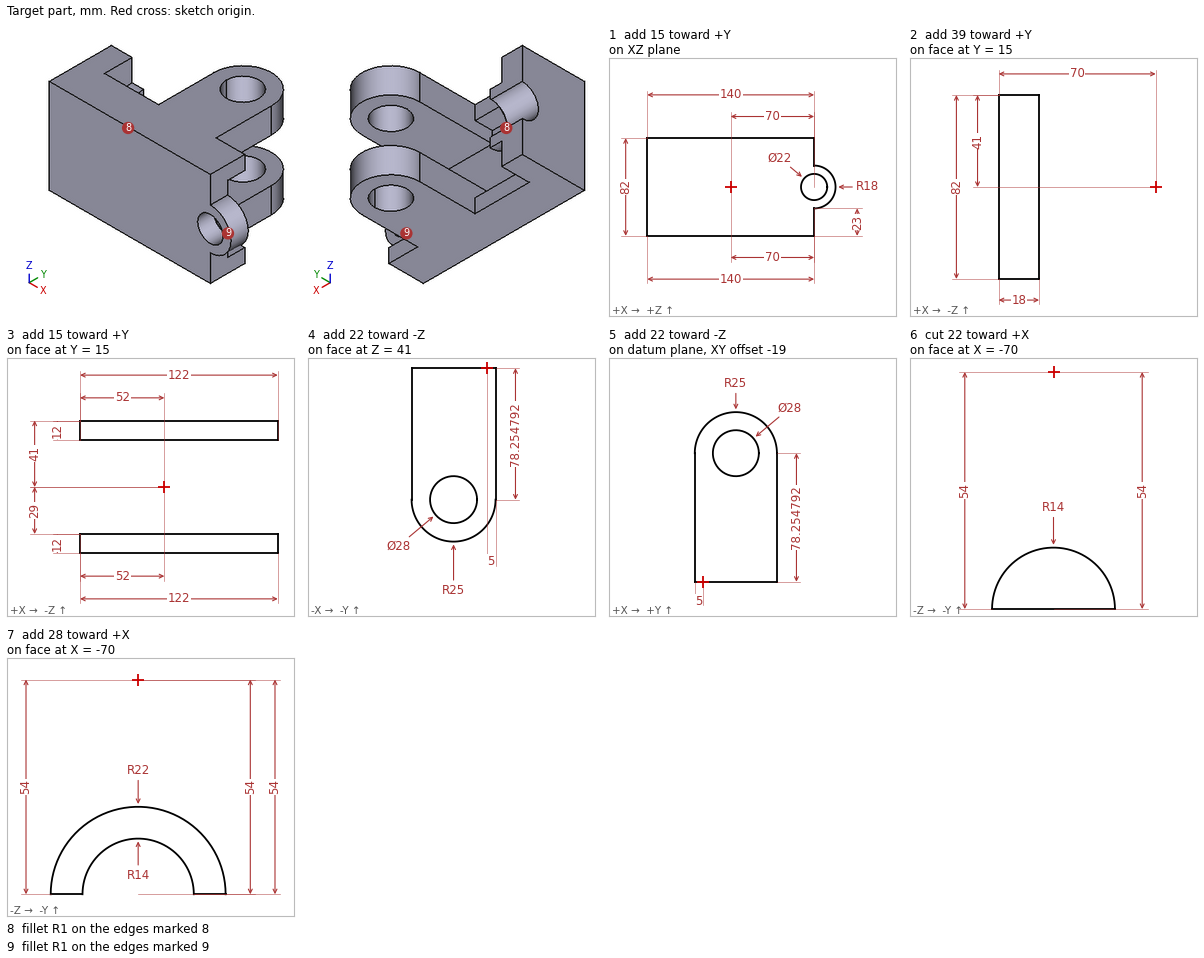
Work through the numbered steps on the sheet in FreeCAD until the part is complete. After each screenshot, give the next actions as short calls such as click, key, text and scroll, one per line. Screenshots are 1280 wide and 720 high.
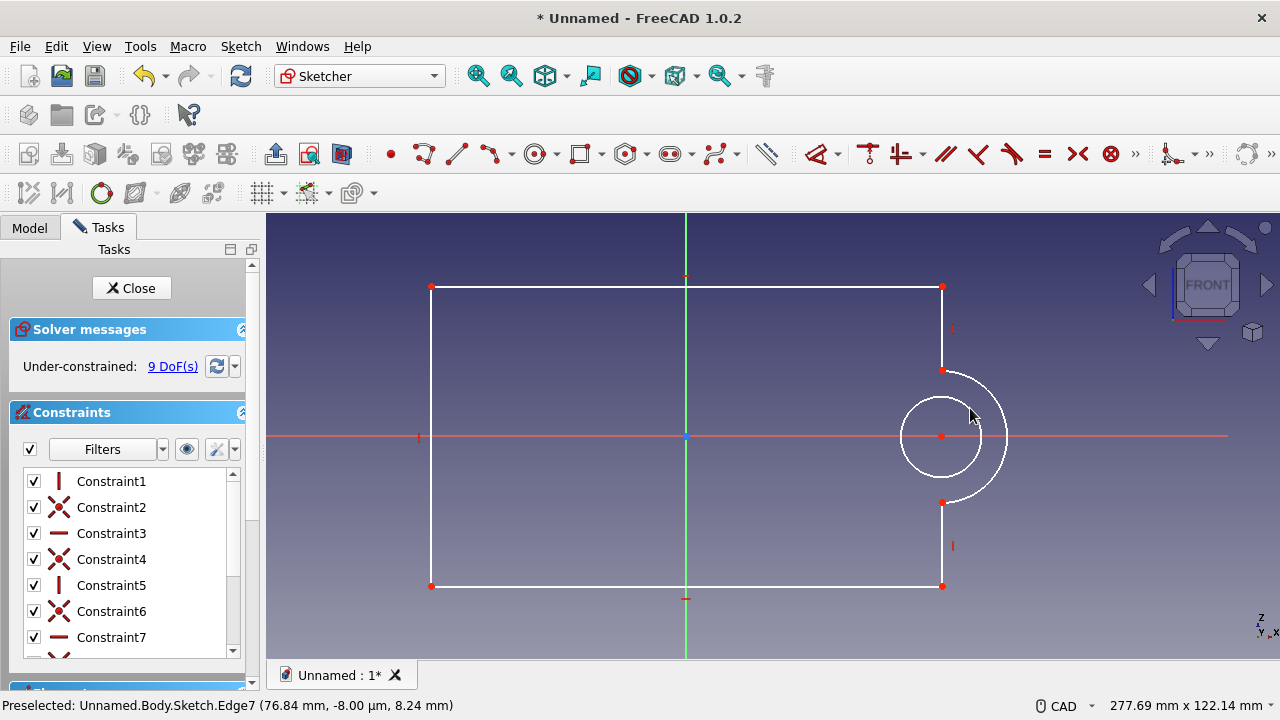
click(941, 437)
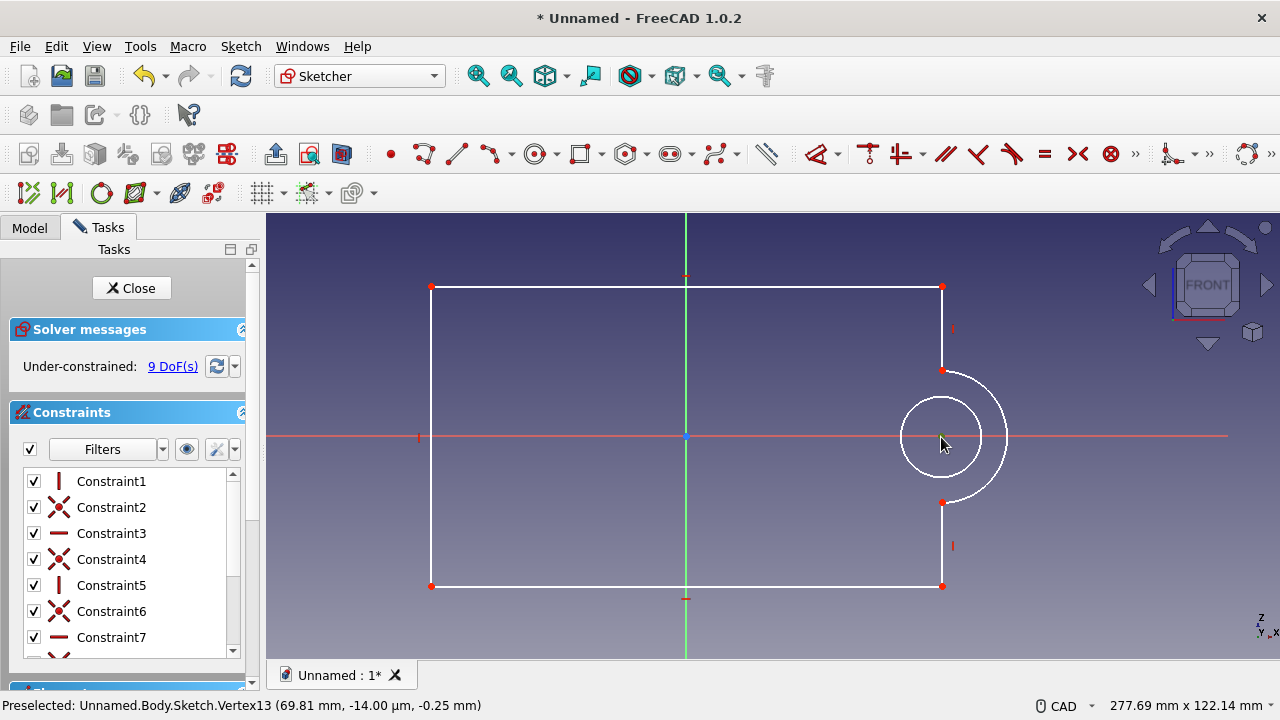
click(353, 436)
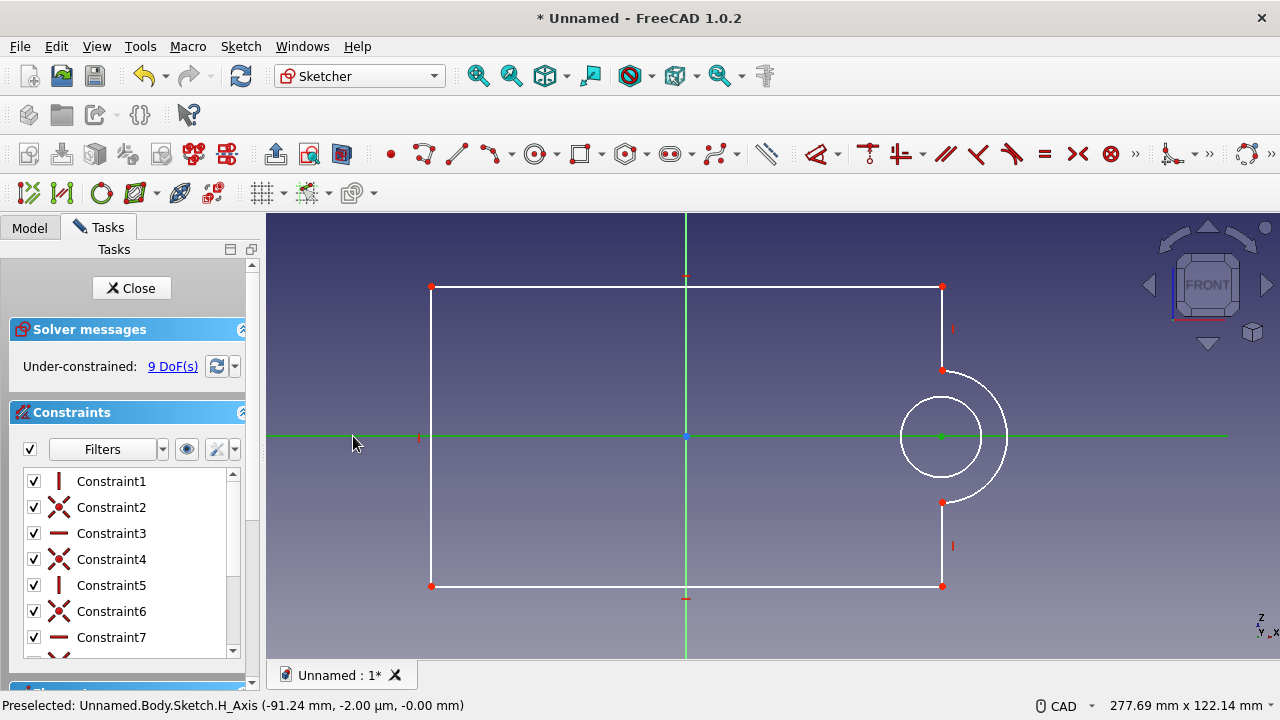
click(868, 154)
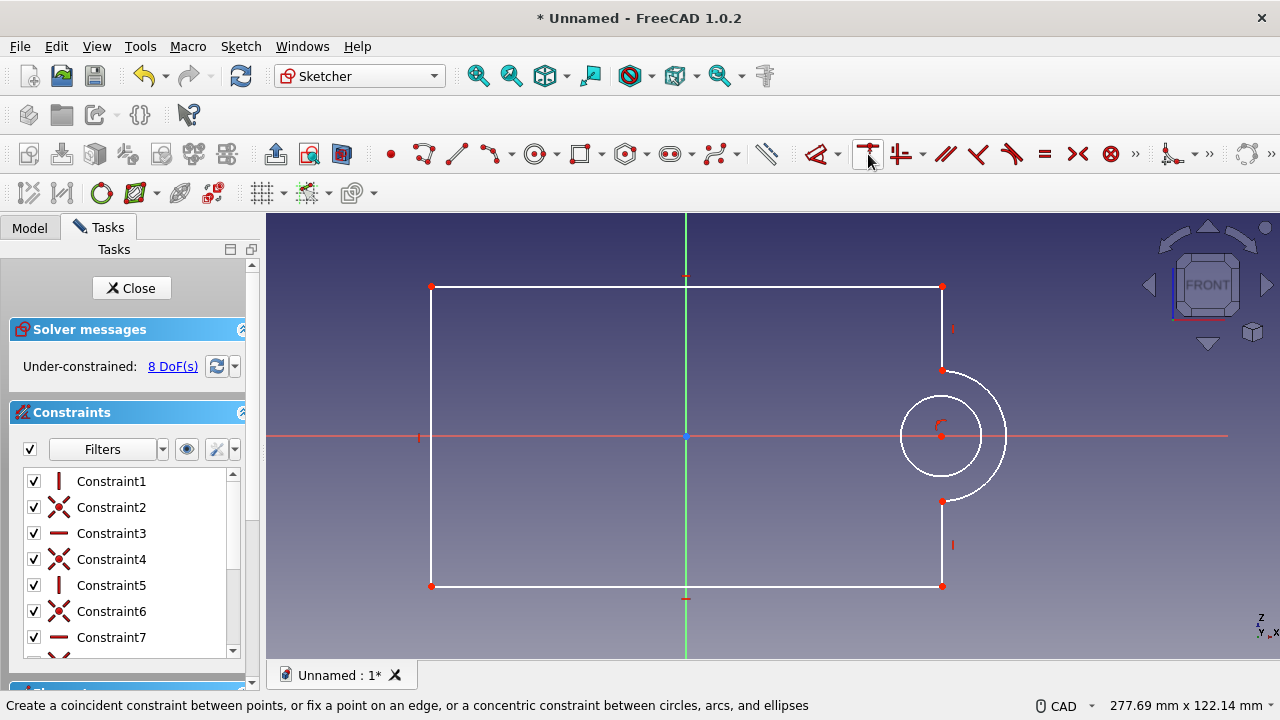
click(816, 154)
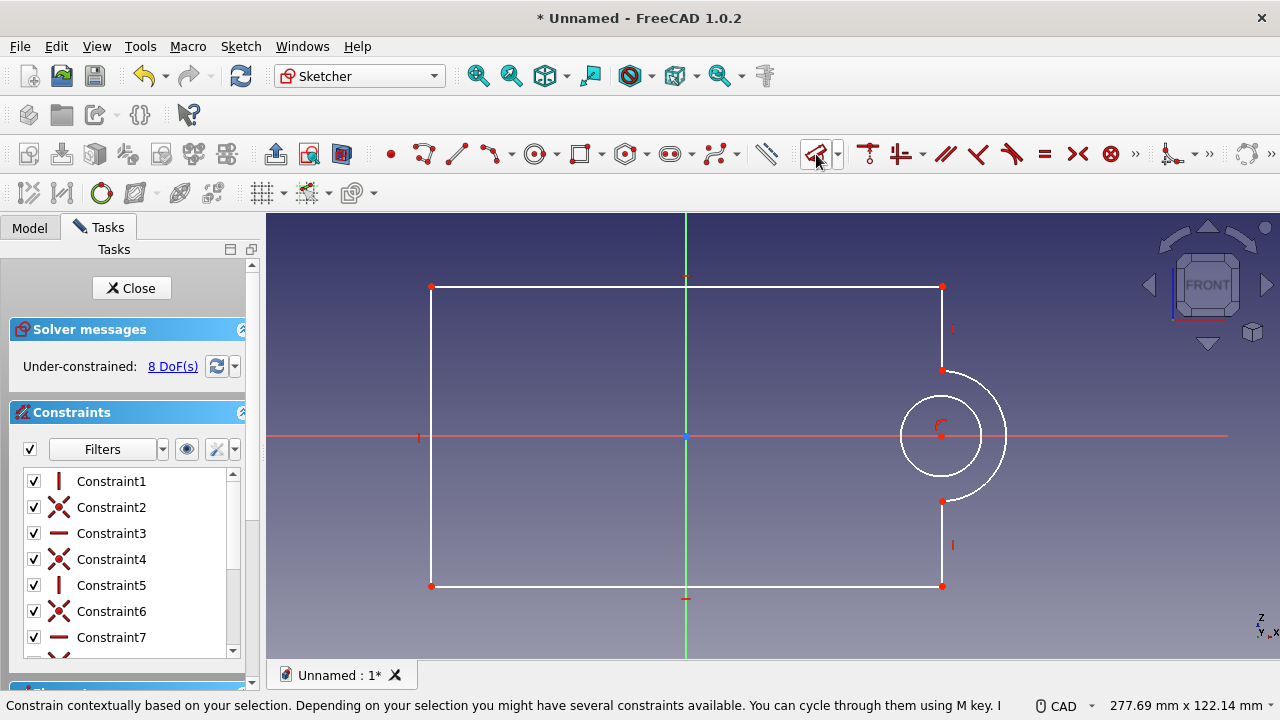
click(994, 474)
click(1020, 493)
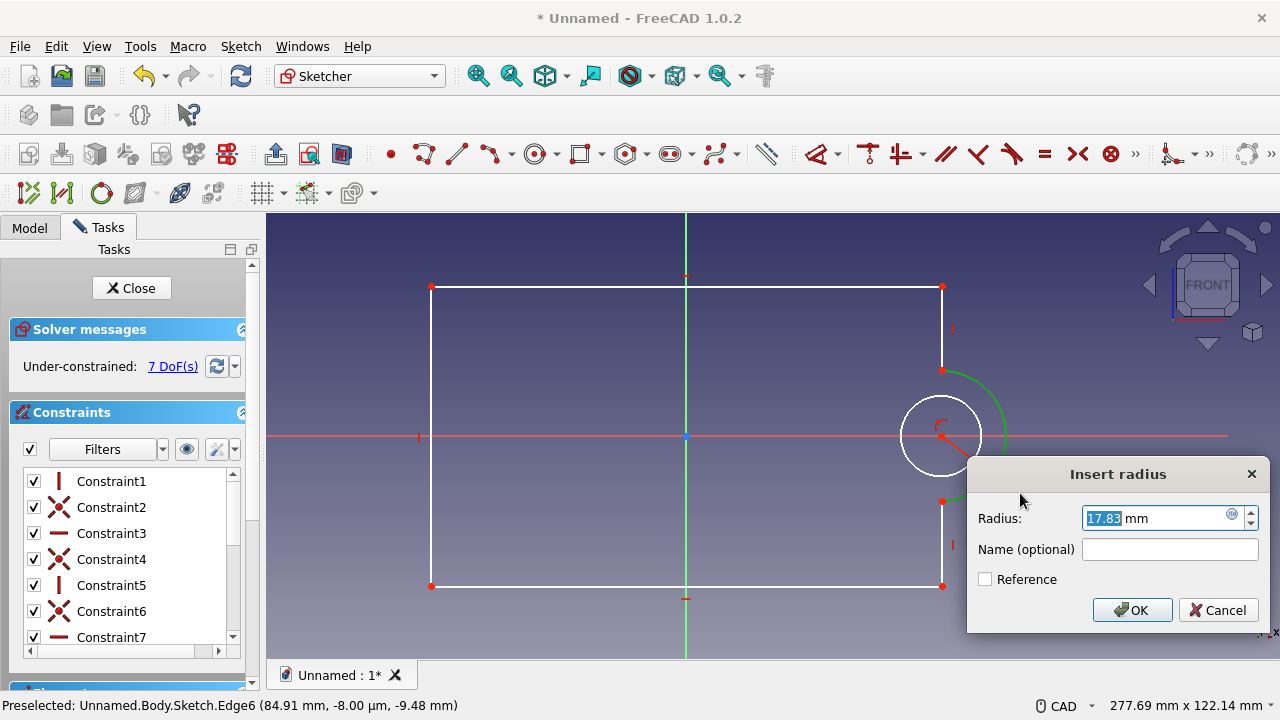
text(18)
key(Return)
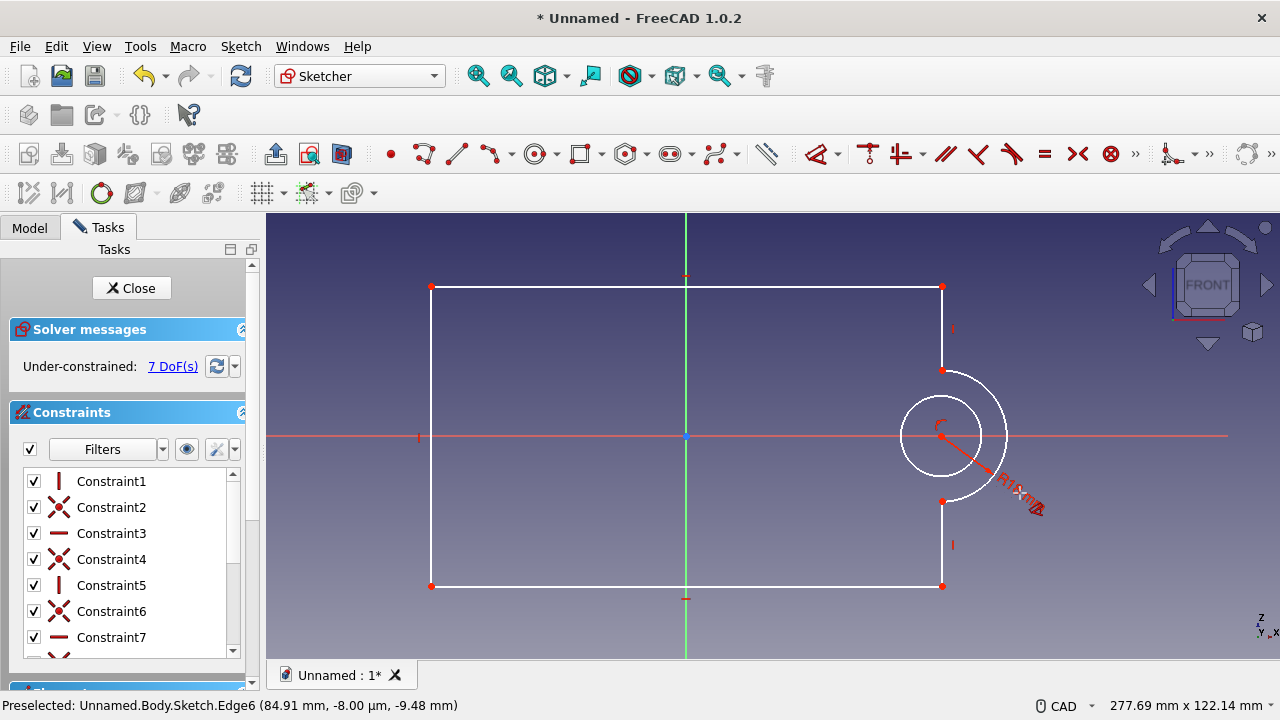
click(969, 408)
click(926, 366)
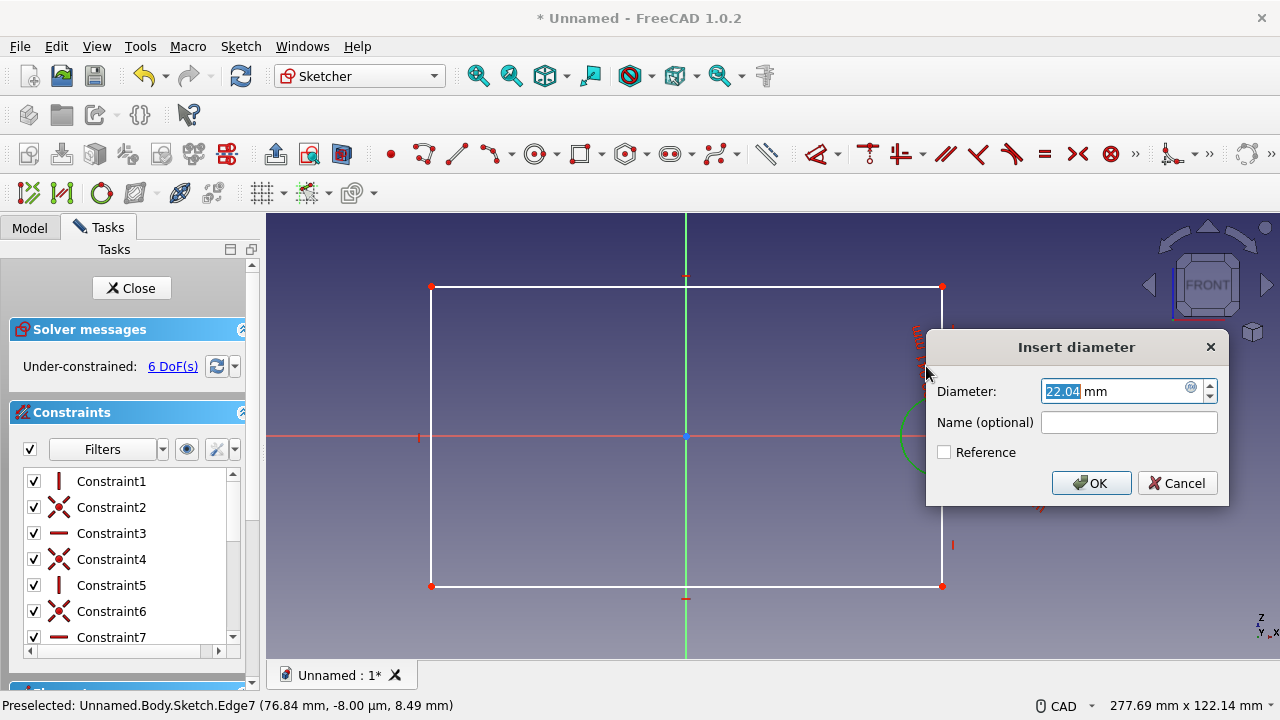
text(22)
key(Return)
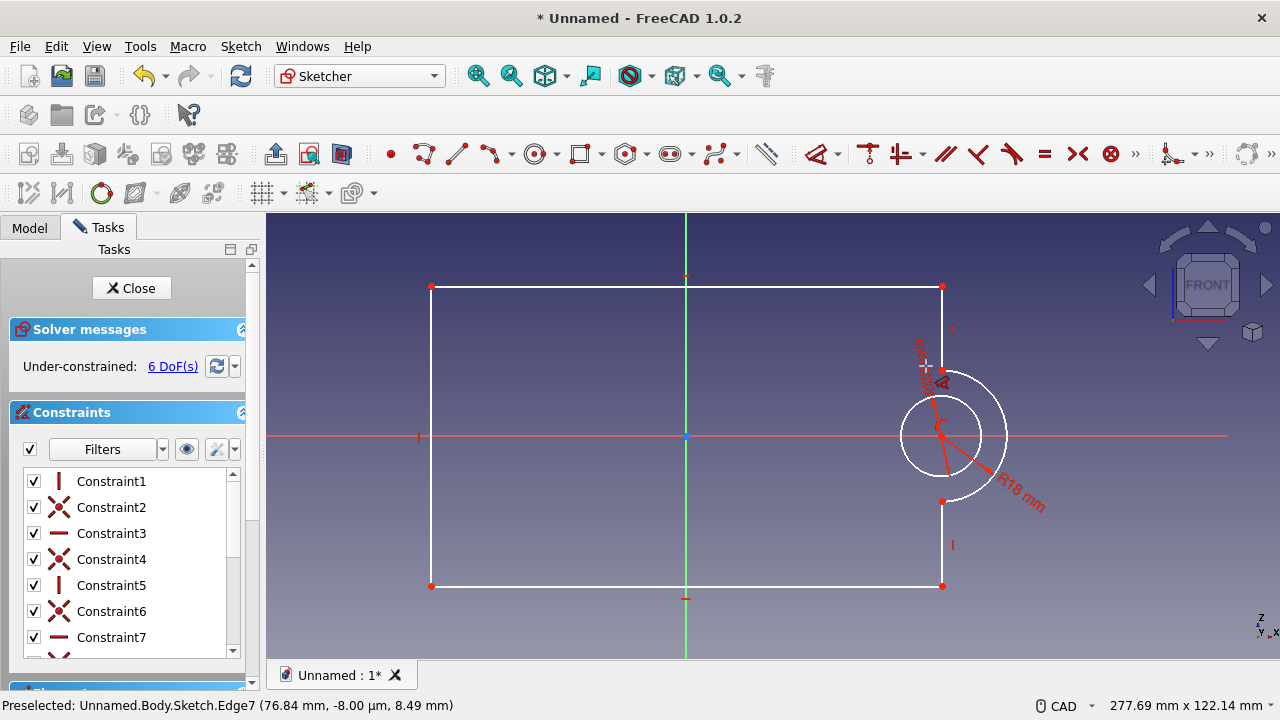
click(942, 527)
click(976, 544)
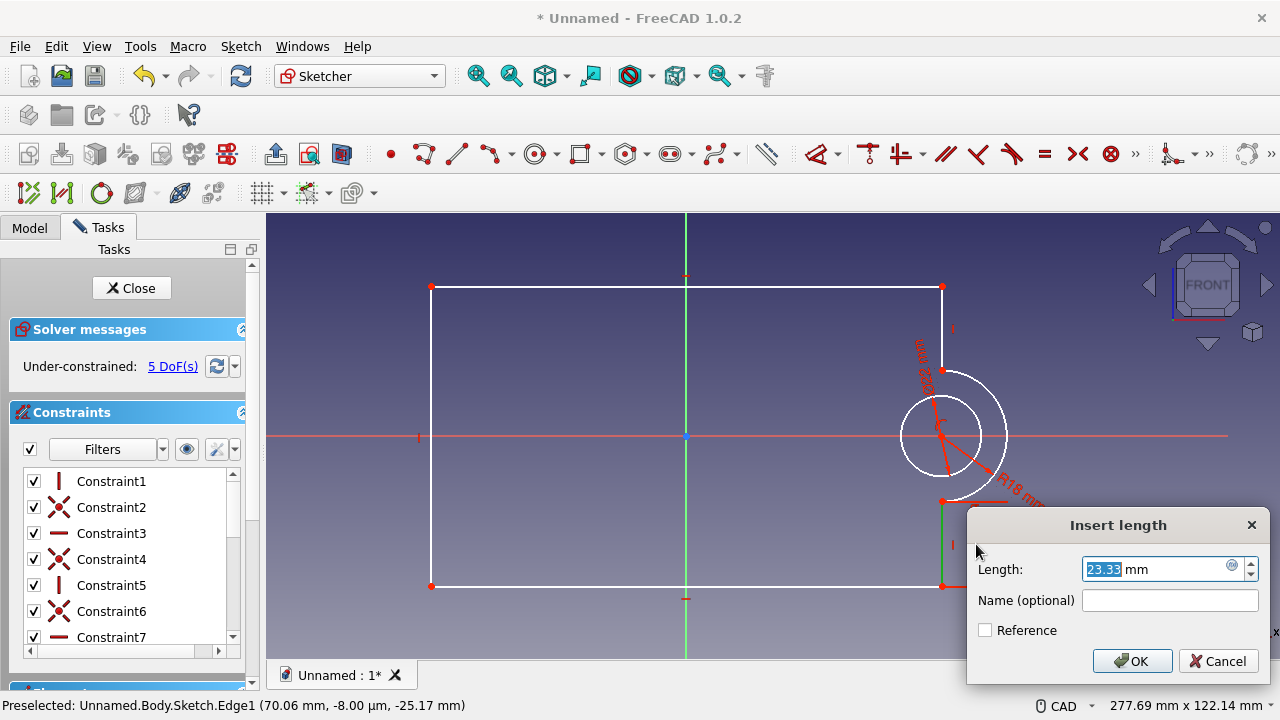
text(23)
key(Return)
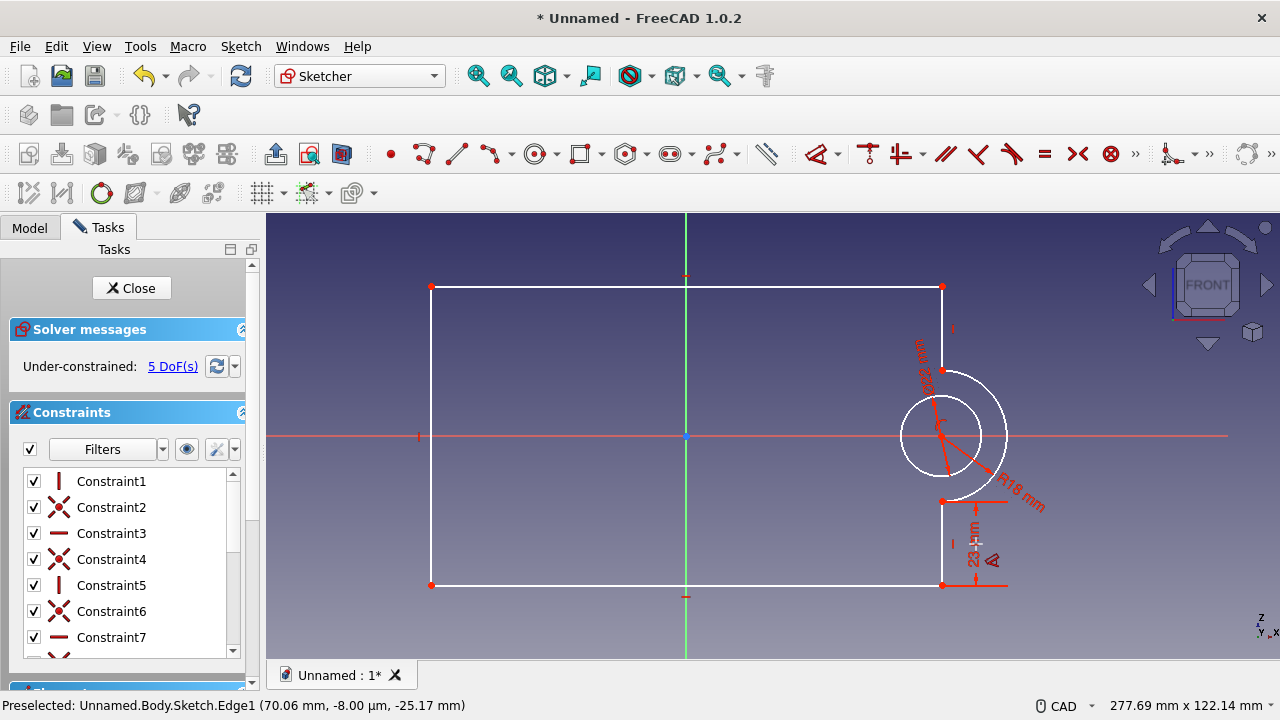
click(431, 496)
click(397, 368)